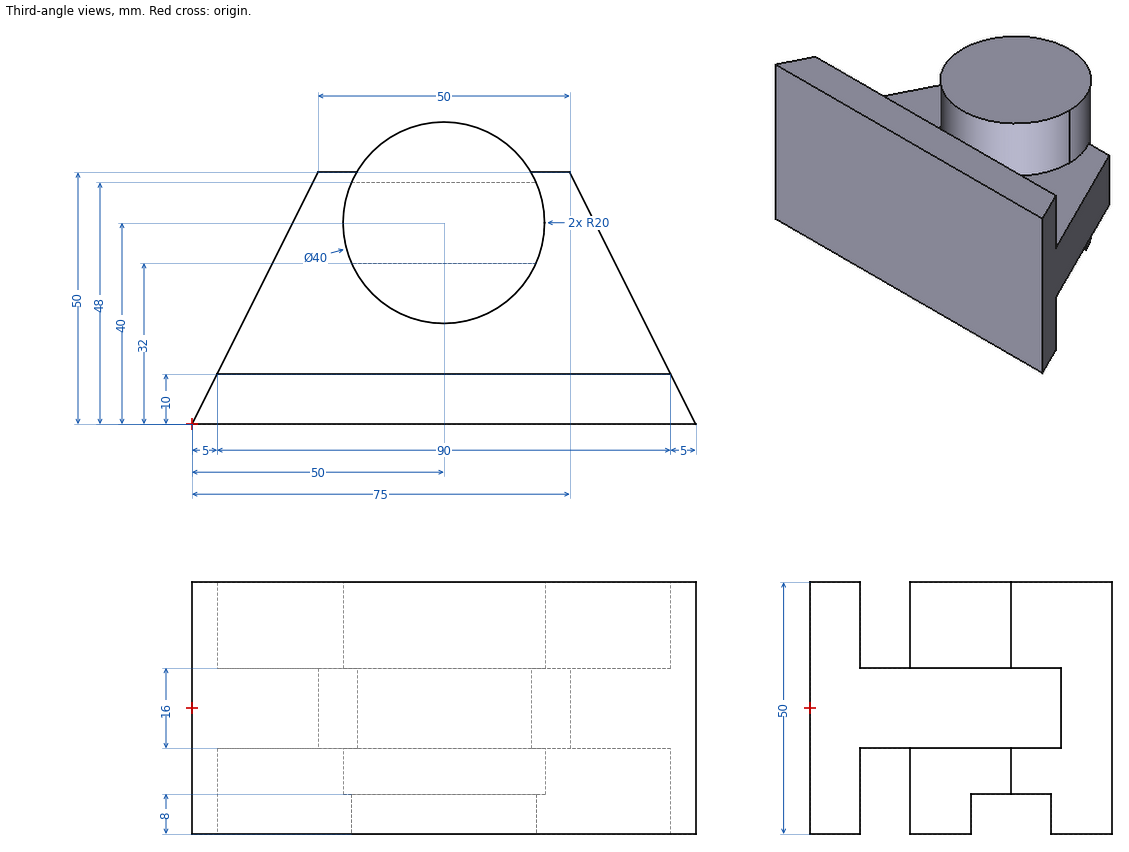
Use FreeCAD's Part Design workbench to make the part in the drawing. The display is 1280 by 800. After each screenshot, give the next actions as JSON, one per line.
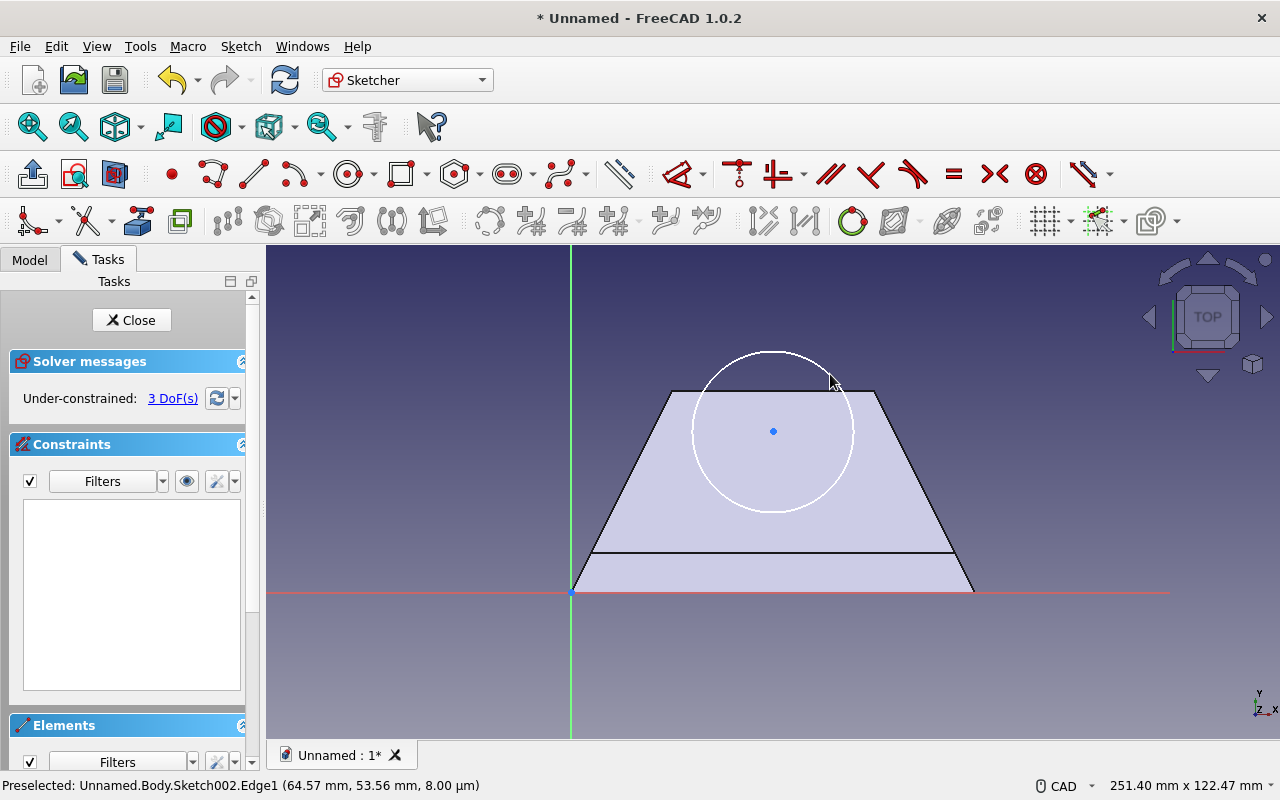
{"action": "left_click", "coordinate": [676, 174]}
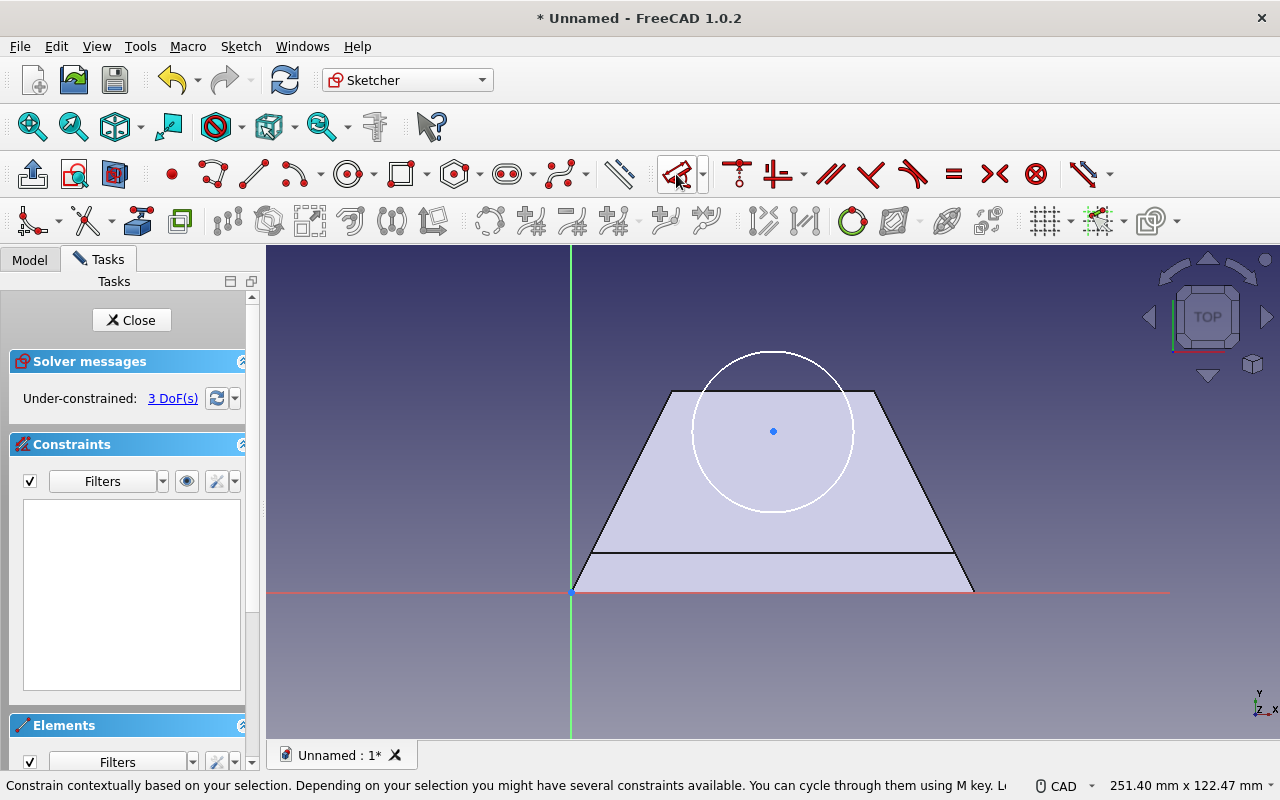
{"action": "left_click", "coordinate": [830, 375]}
{"action": "left_click", "coordinate": [853, 352]}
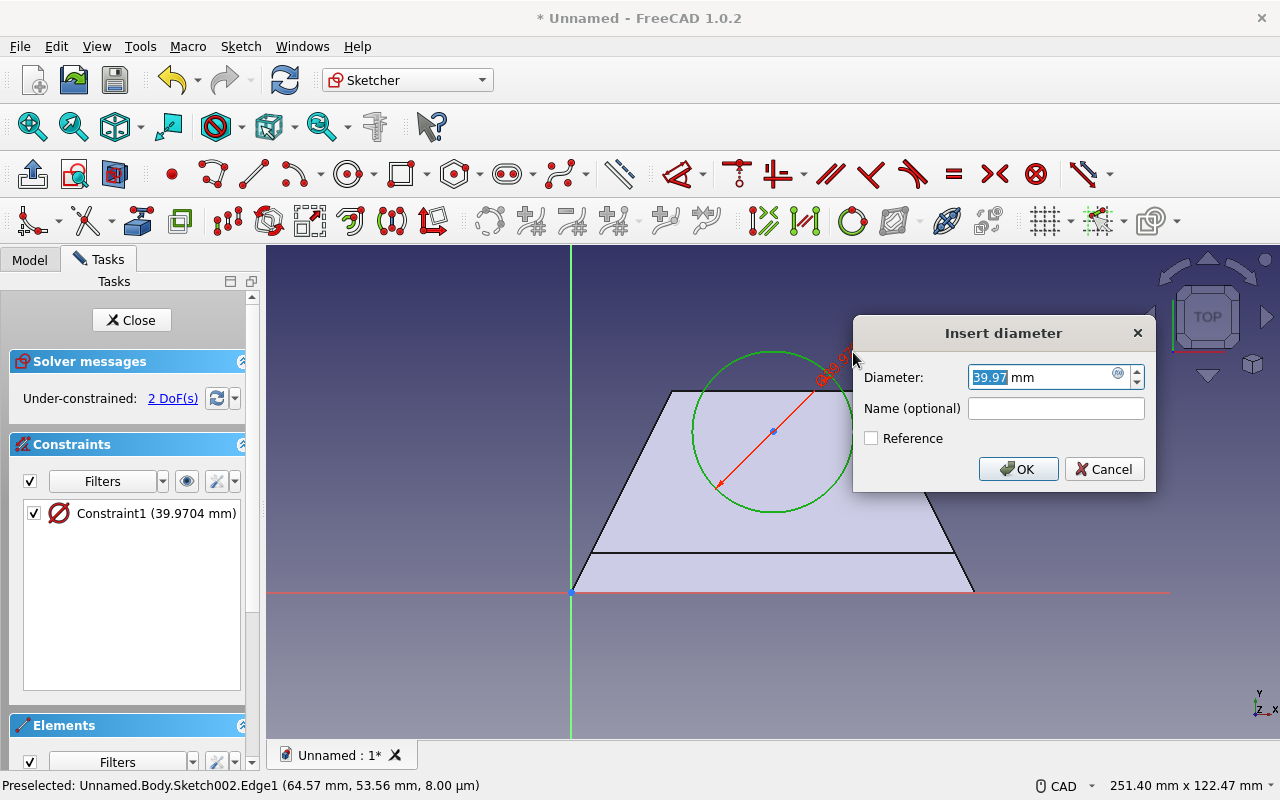
{"action": "type", "text": "40"}
{"action": "key", "text": "Return"}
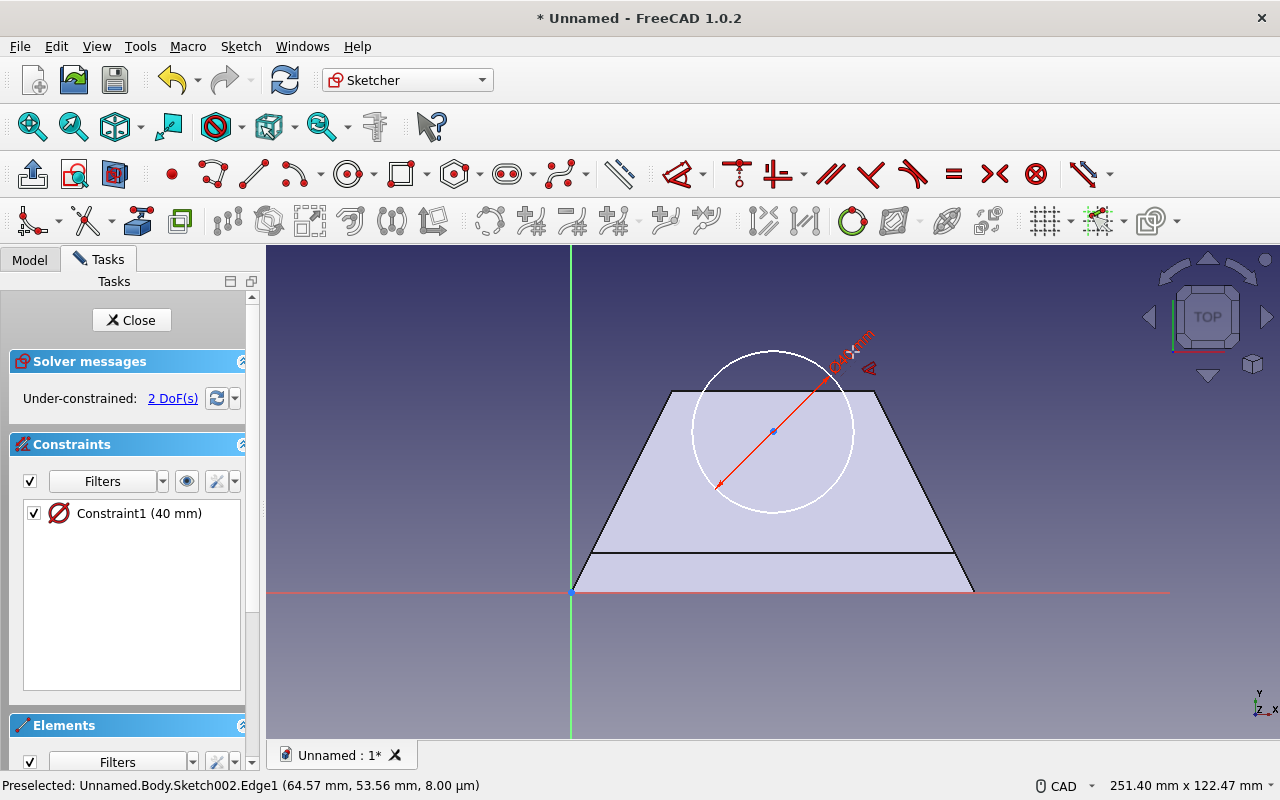
{"action": "left_click", "coordinate": [773, 432]}
{"action": "left_click", "coordinate": [672, 627]}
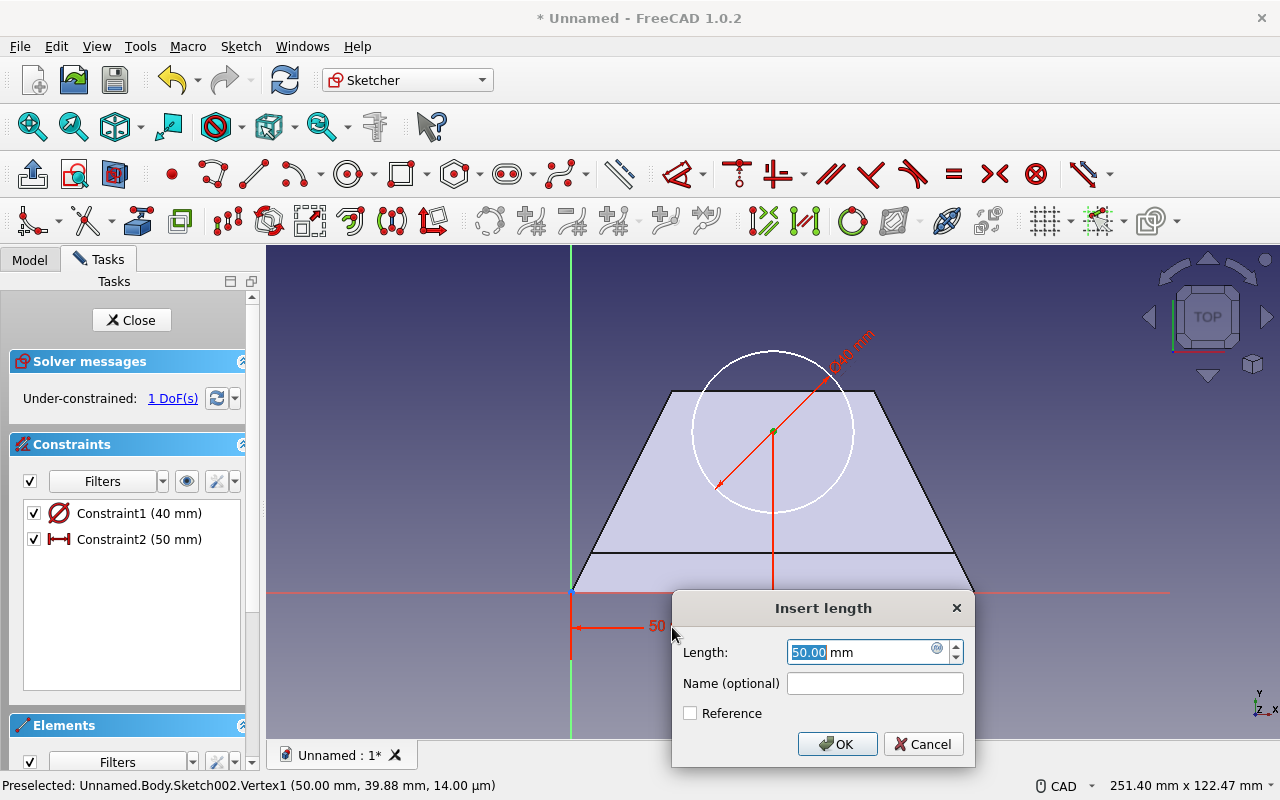
{"action": "type", "text": "50"}
{"action": "key", "text": "Return"}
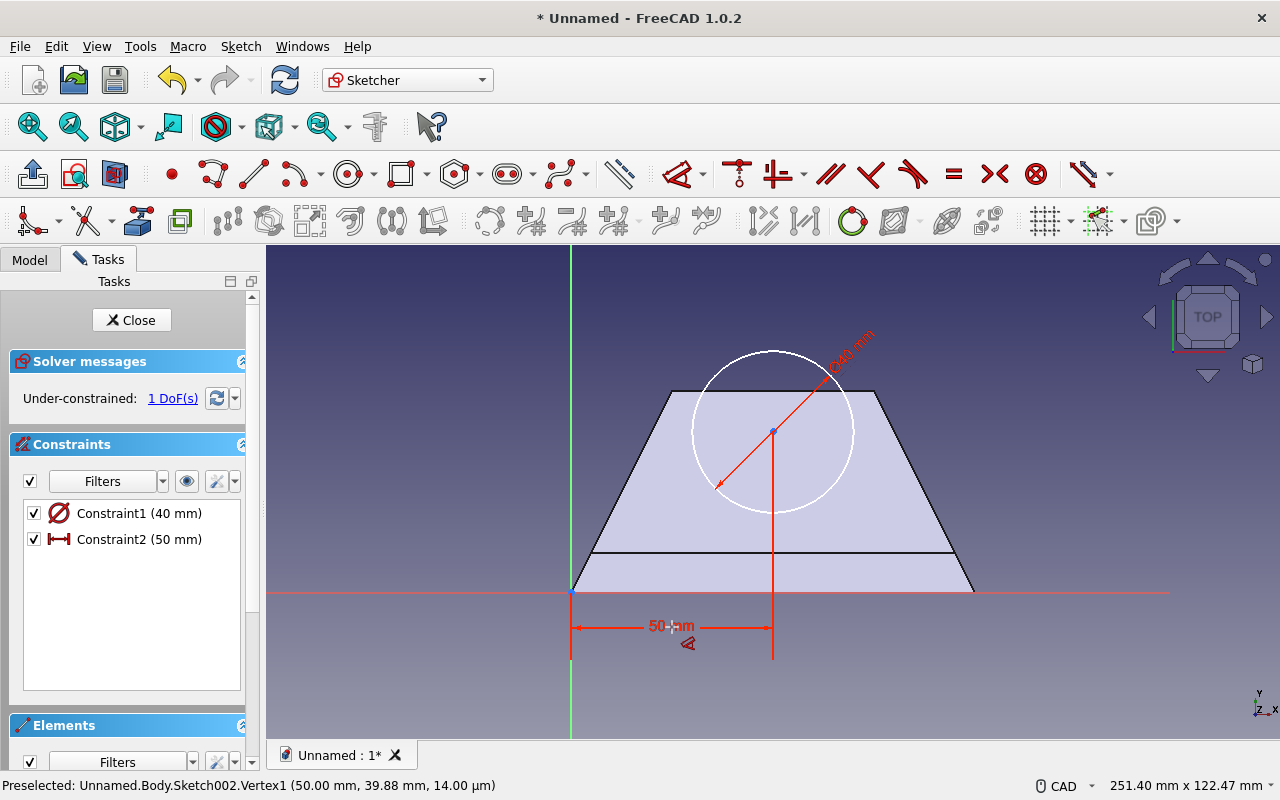
{"action": "left_click", "coordinate": [773, 432]}
{"action": "left_click", "coordinate": [537, 512]}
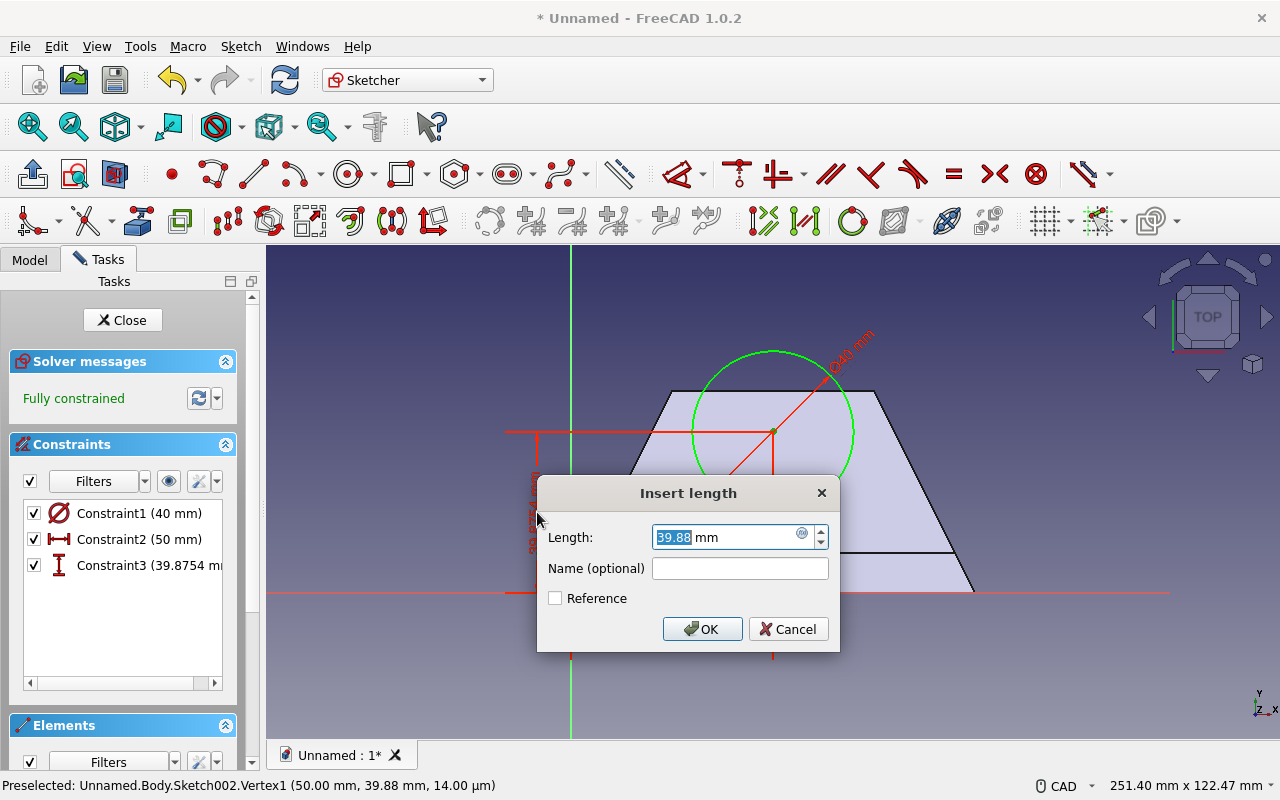
{"action": "type", "text": "40"}
{"action": "key", "text": "Return"}
{"action": "key", "text": "Escape"}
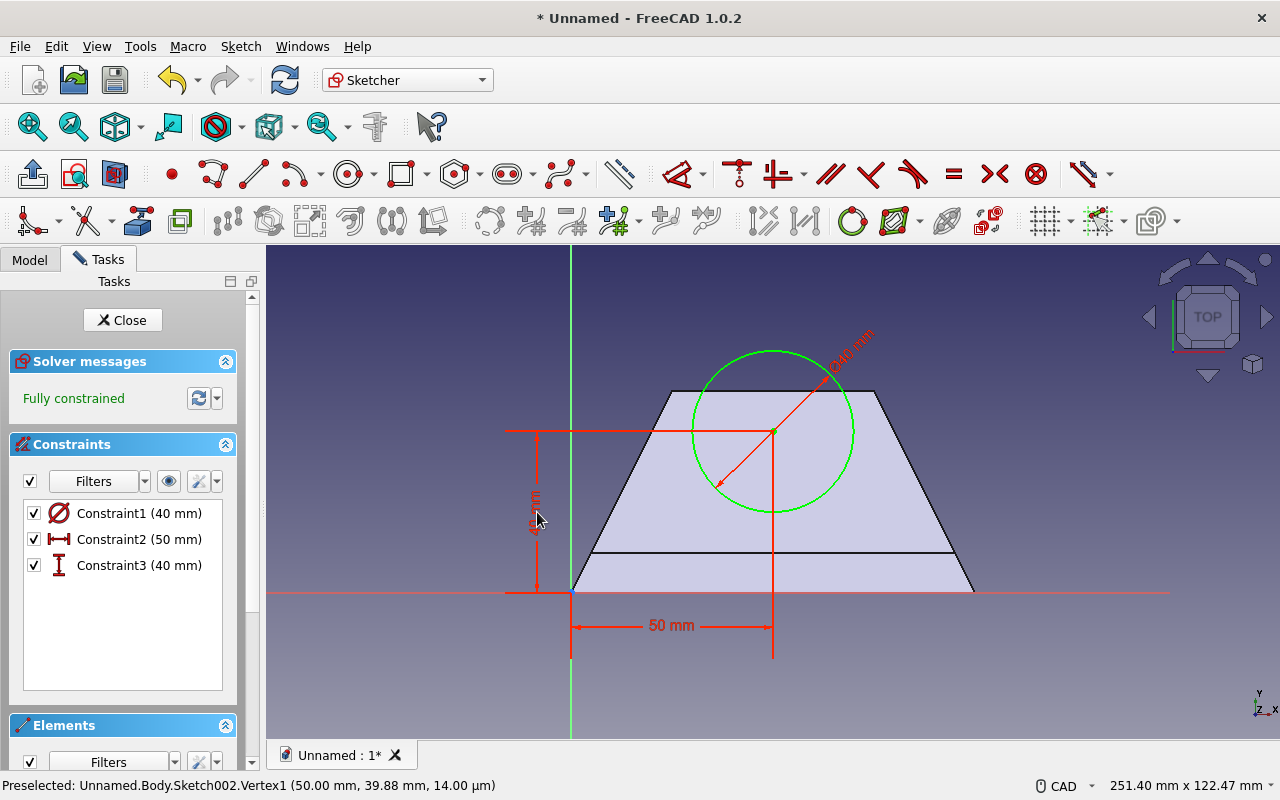
{"action": "left_click", "coordinate": [123, 320]}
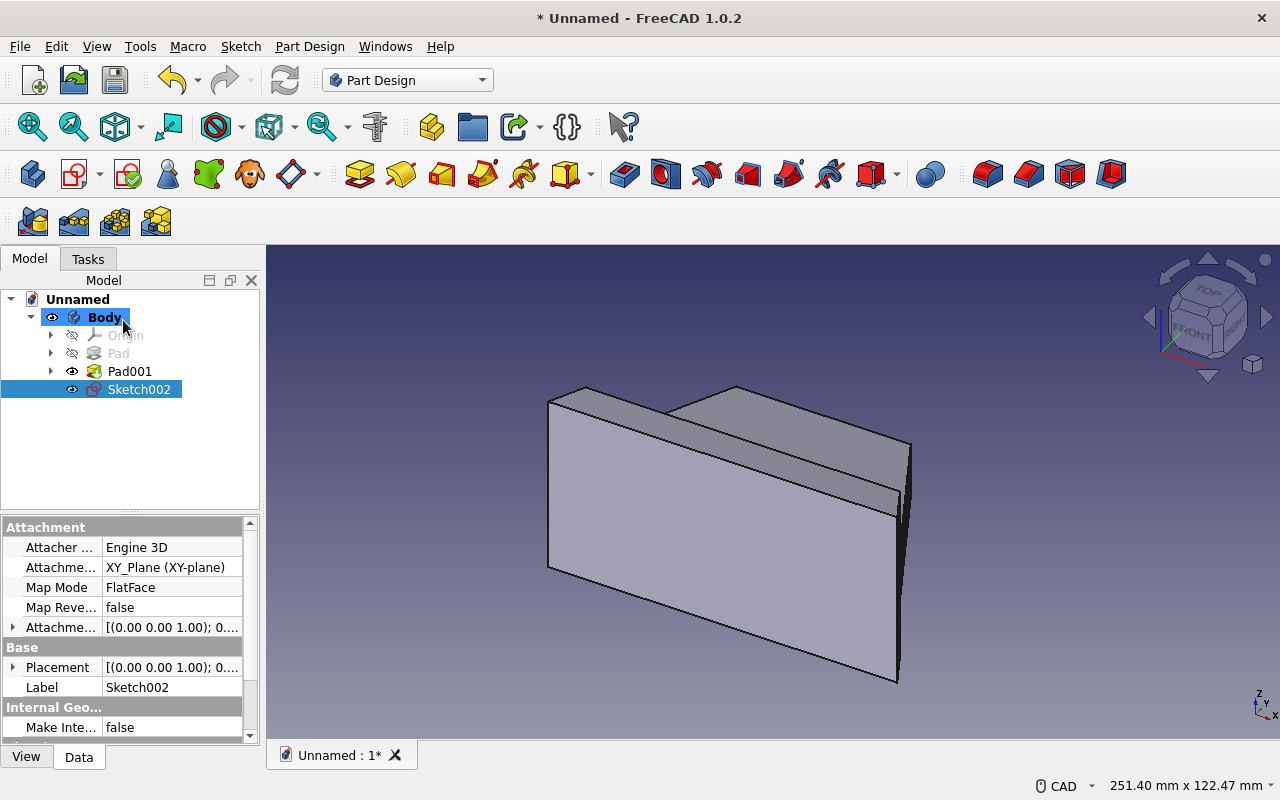
{"action": "left_click", "coordinate": [360, 174]}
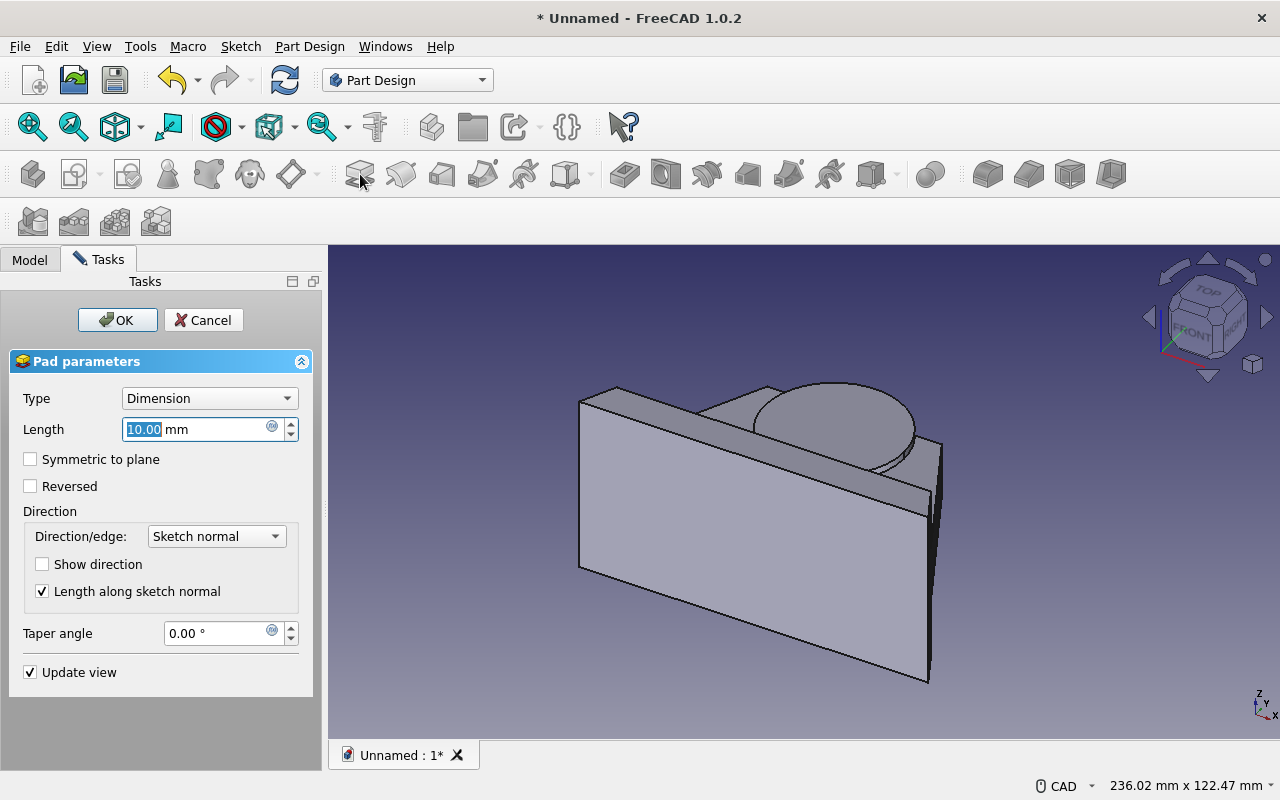
{"action": "type", "text": "50"}
{"action": "key", "text": "Tab"}